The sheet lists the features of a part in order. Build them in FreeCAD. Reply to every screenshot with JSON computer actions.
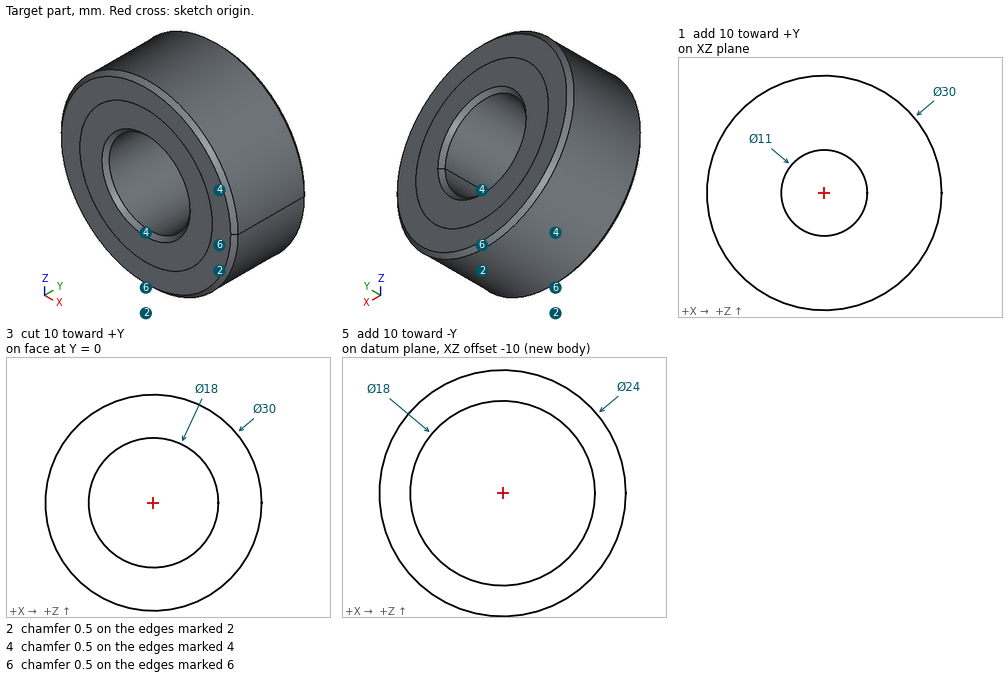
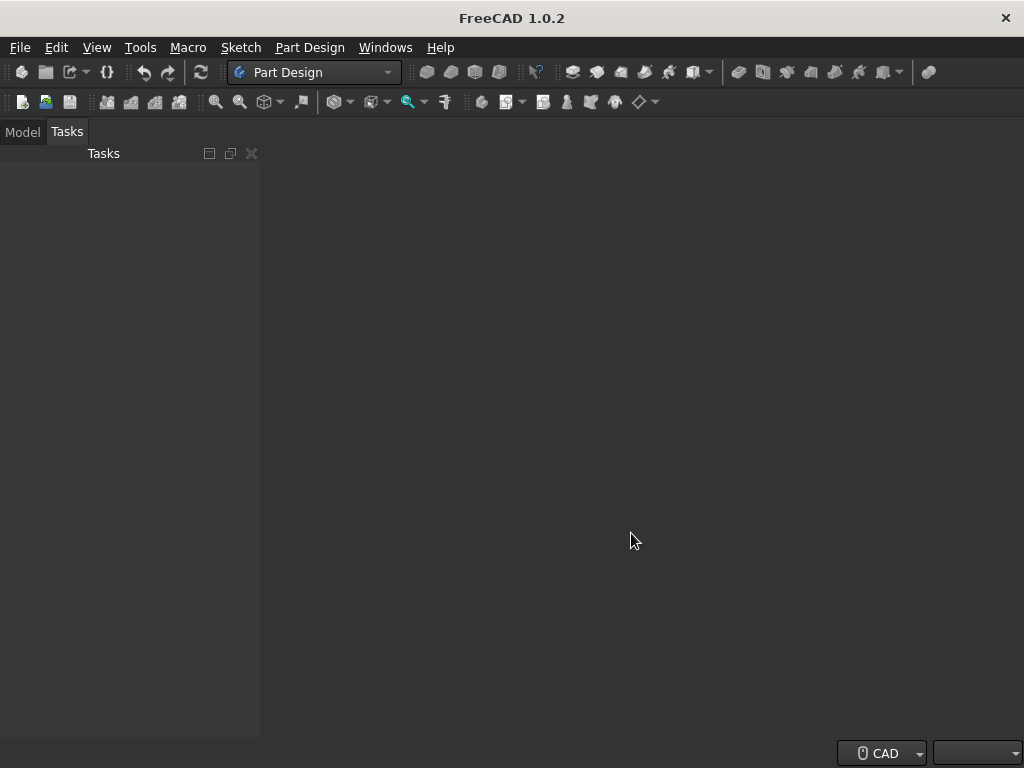
{"action": "left_click", "coordinate": [22, 102]}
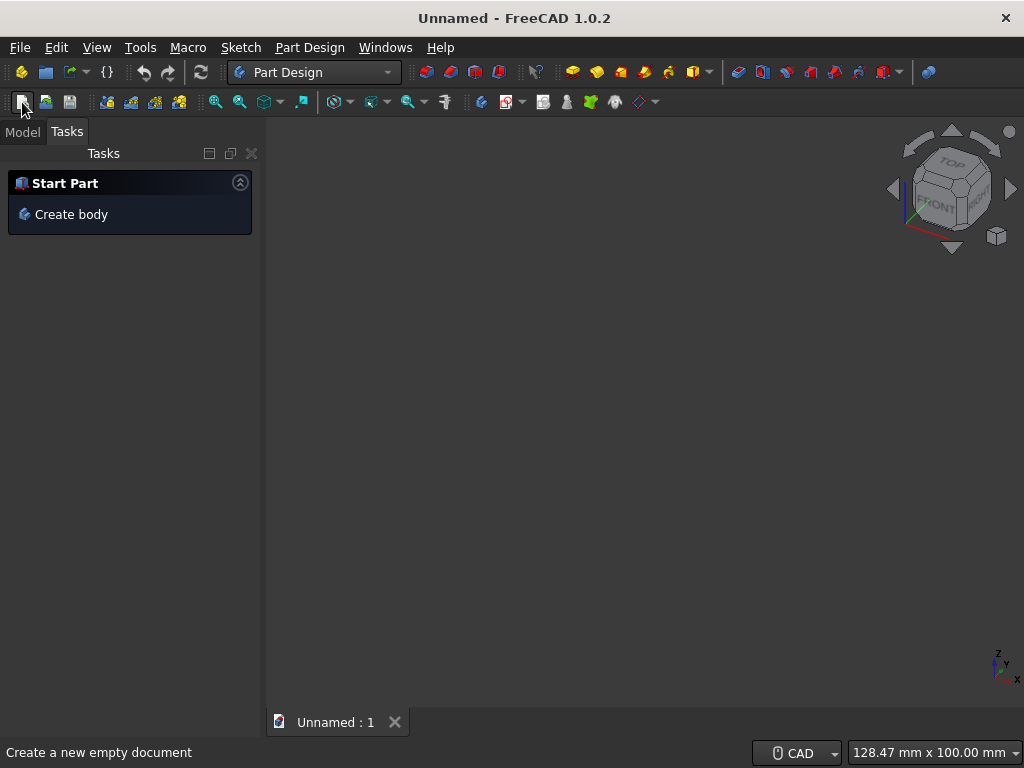
{"action": "left_click", "coordinate": [506, 102]}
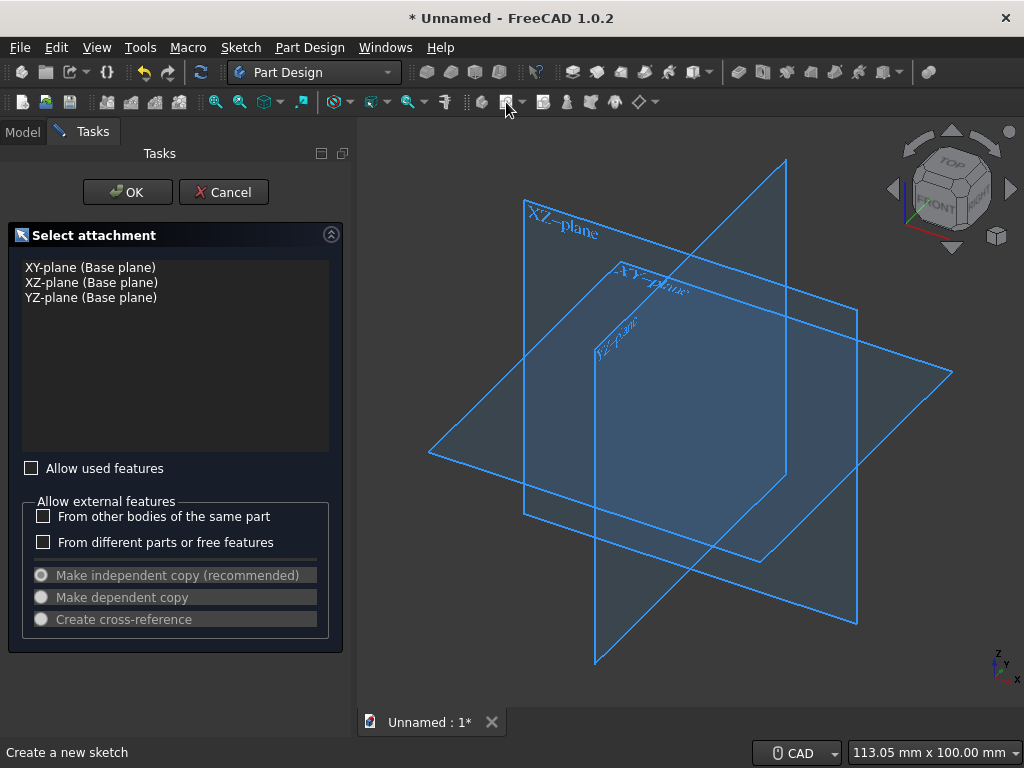
{"action": "left_click", "coordinate": [82, 282]}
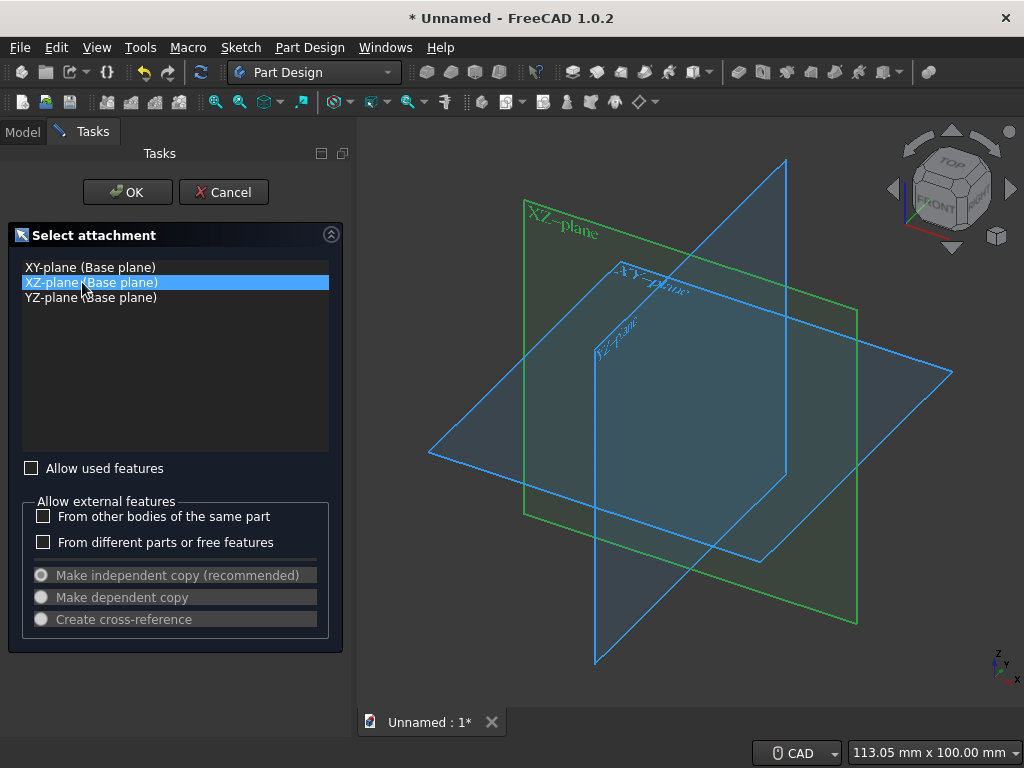
{"action": "left_click", "coordinate": [128, 192]}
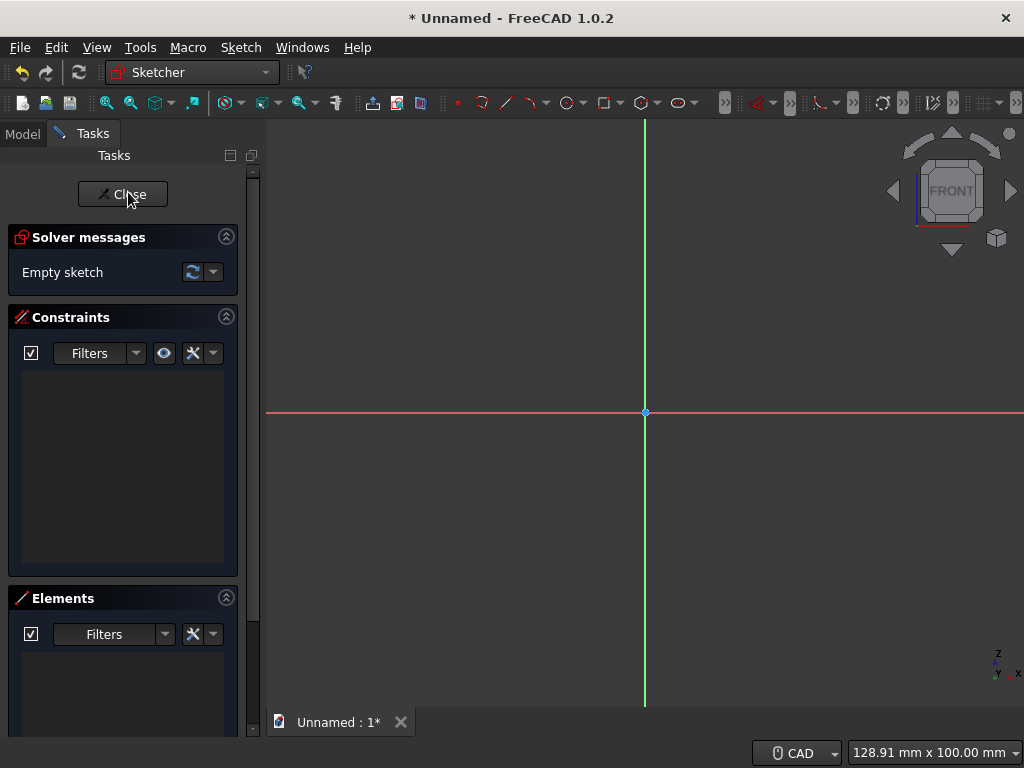
{"action": "scroll", "coordinate": [701, 413], "scroll_direction": "up", "scroll_amount": 4}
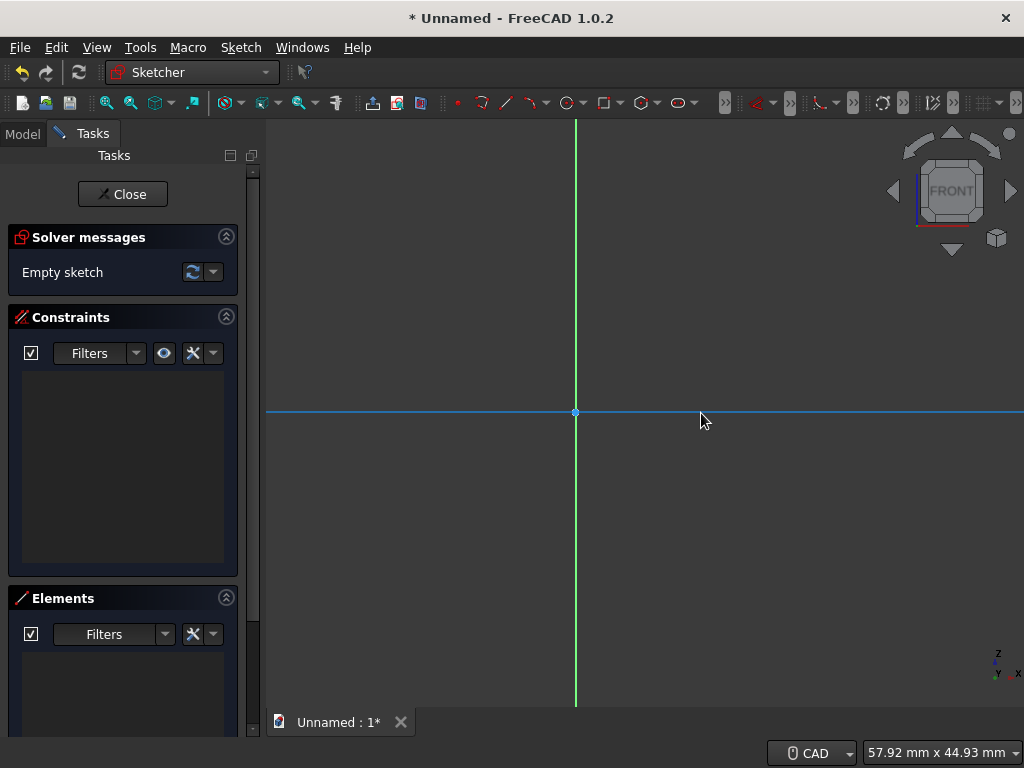
{"action": "left_click", "coordinate": [568, 104]}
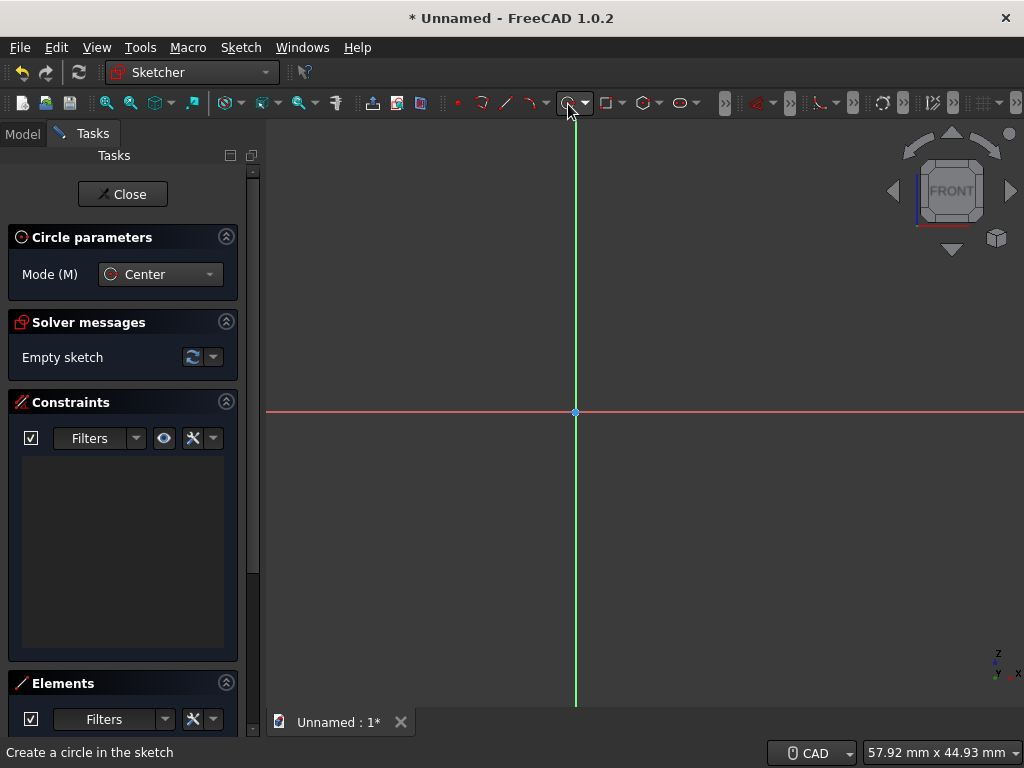
{"action": "left_click", "coordinate": [576, 412]}
{"action": "left_click", "coordinate": [714, 274]}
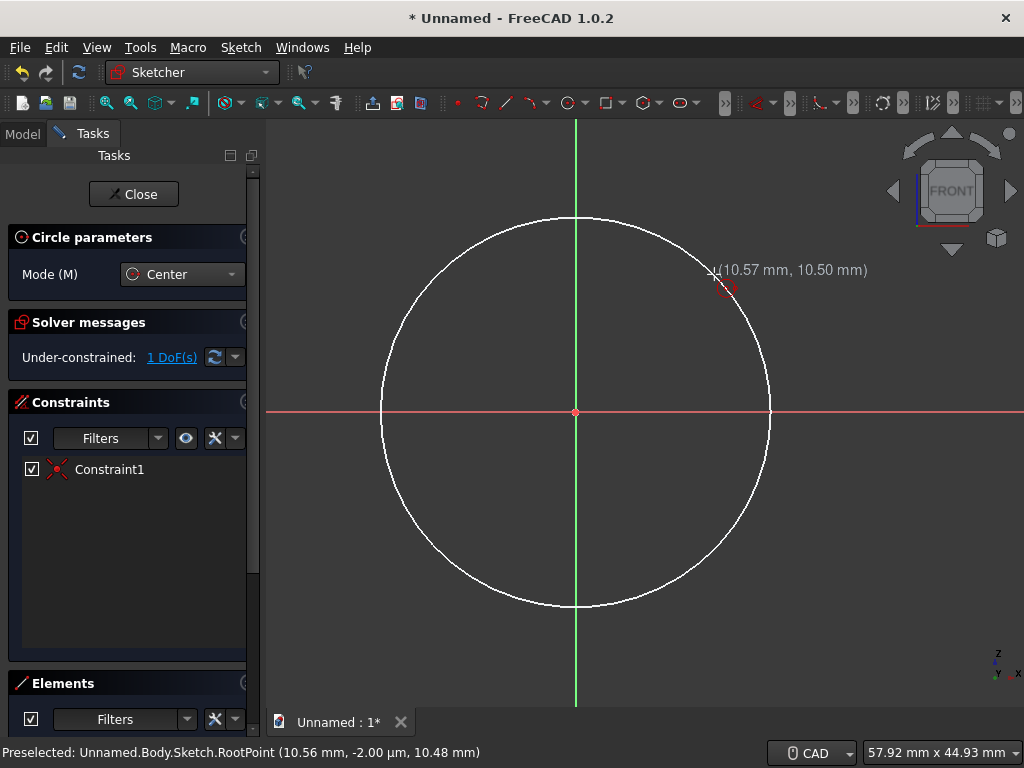
{"action": "left_click", "coordinate": [576, 412]}
{"action": "left_click", "coordinate": [627, 361]}
{"action": "key", "text": "Escape"}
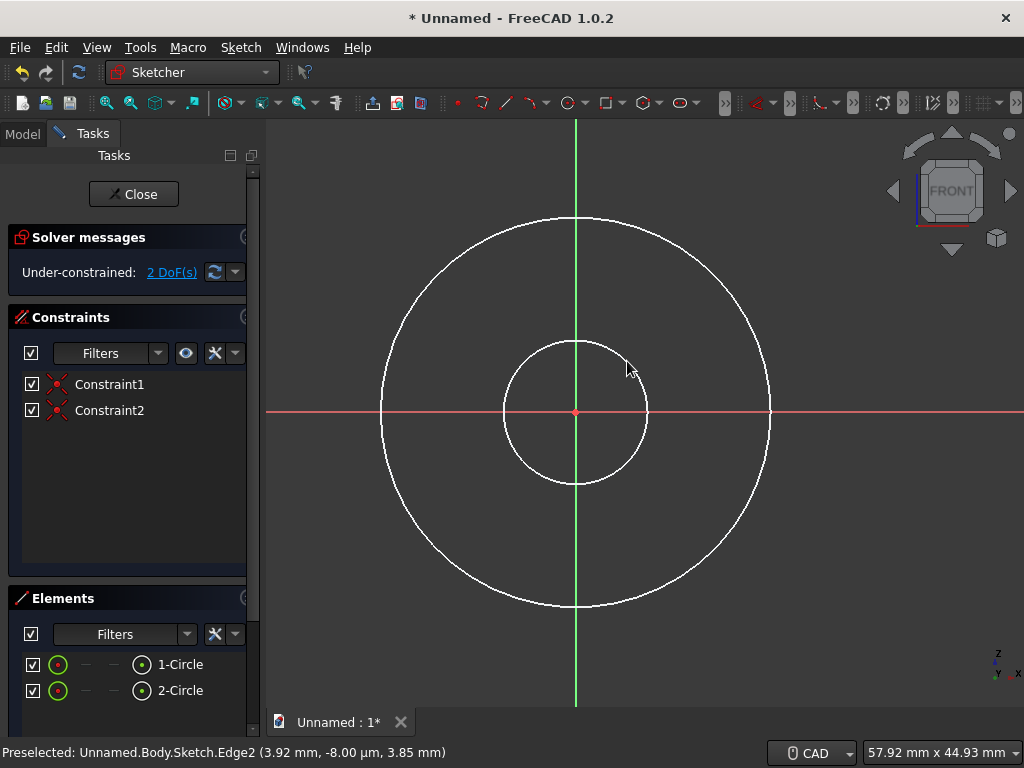
{"action": "left_click", "coordinate": [713, 274]}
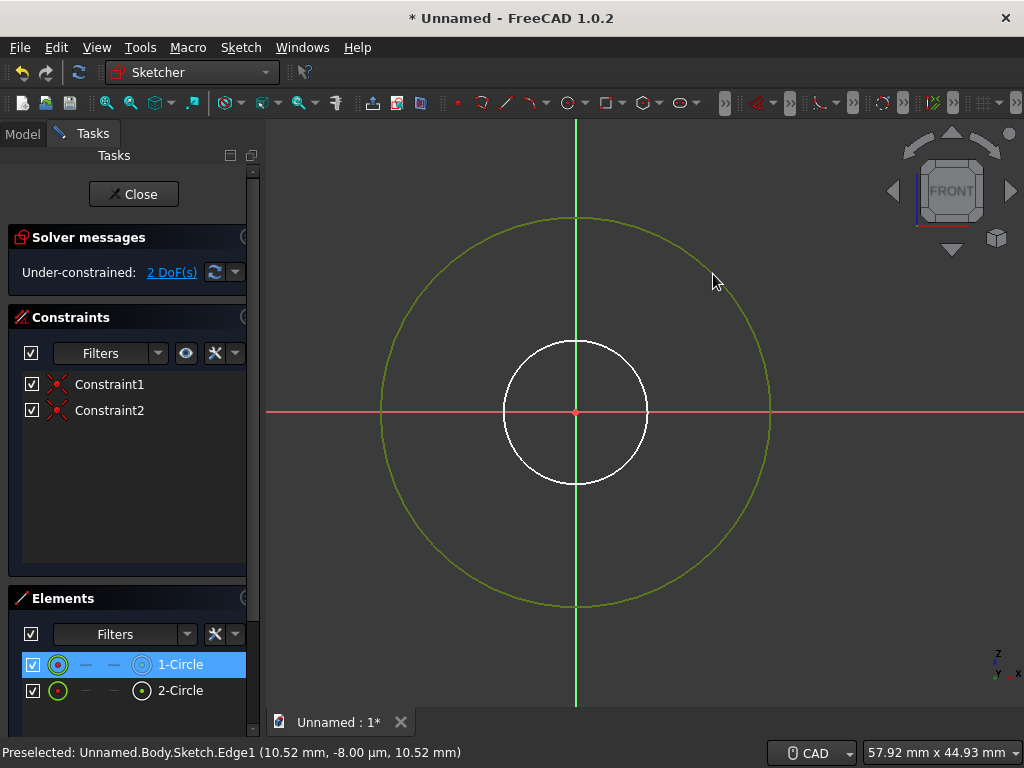
{"action": "key", "text": "k o"}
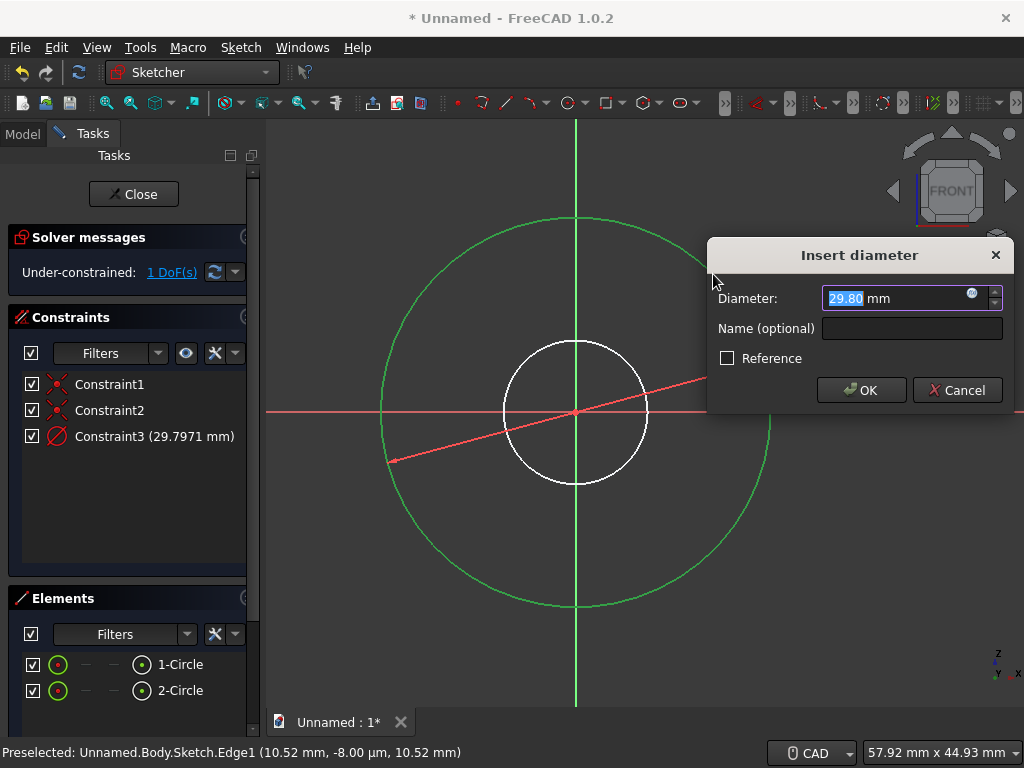
{"action": "type", "text": "30"}
{"action": "key", "text": "Return"}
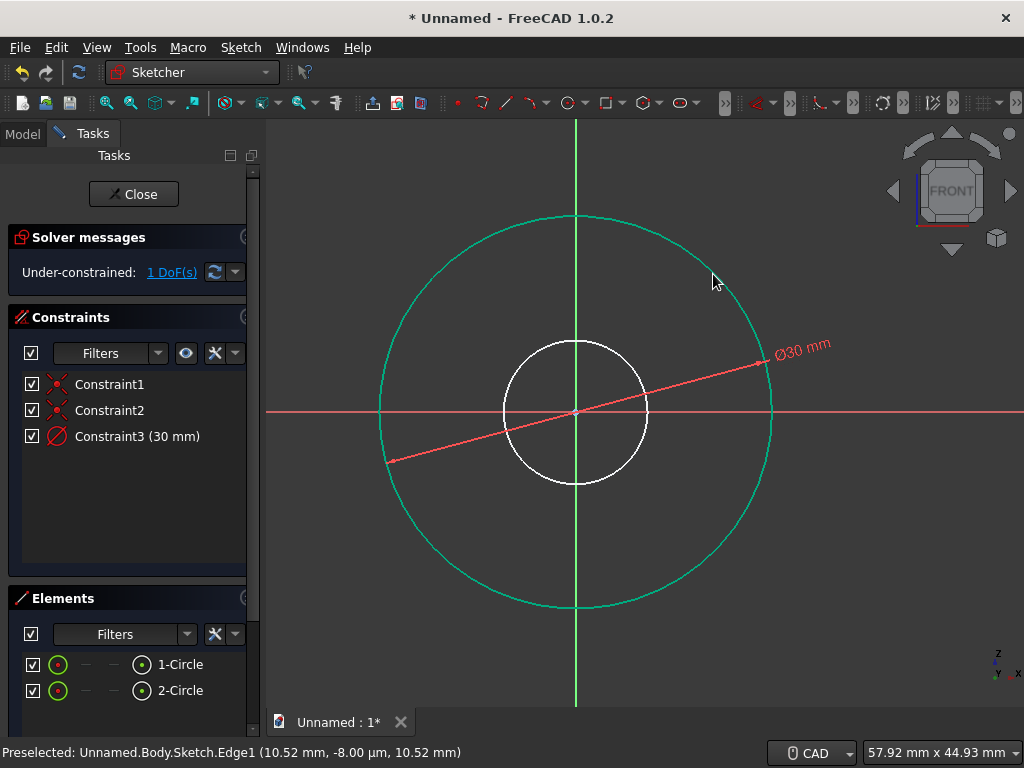
{"action": "left_click", "coordinate": [626, 361]}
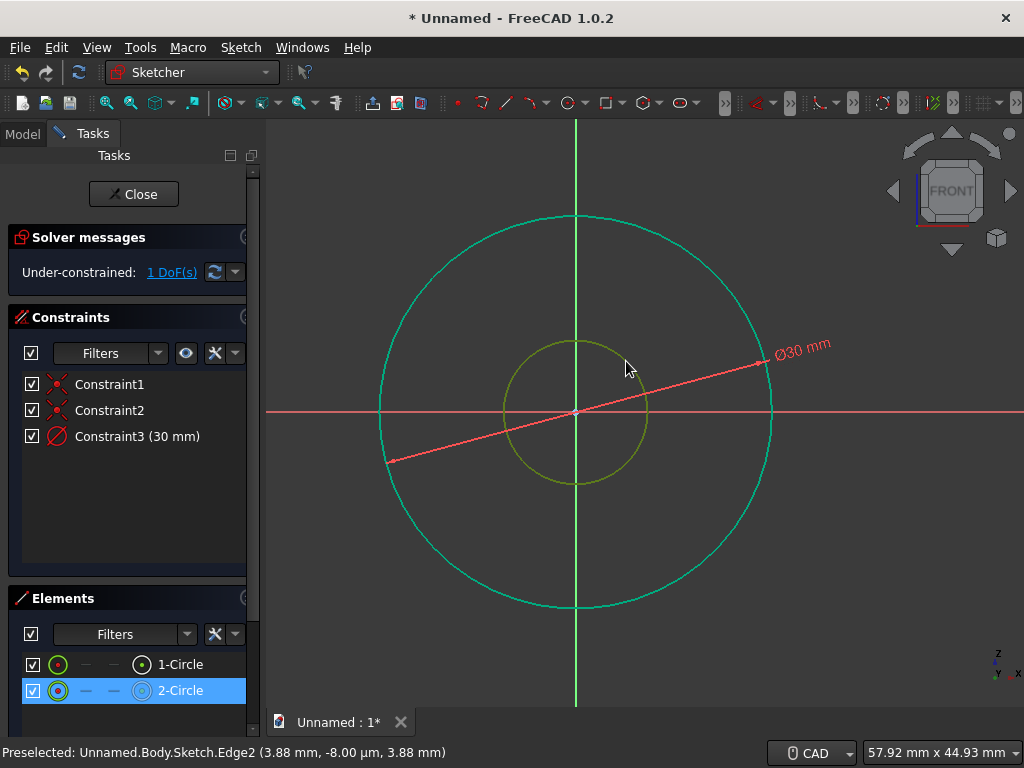
{"action": "left_click", "coordinate": [776, 104]}